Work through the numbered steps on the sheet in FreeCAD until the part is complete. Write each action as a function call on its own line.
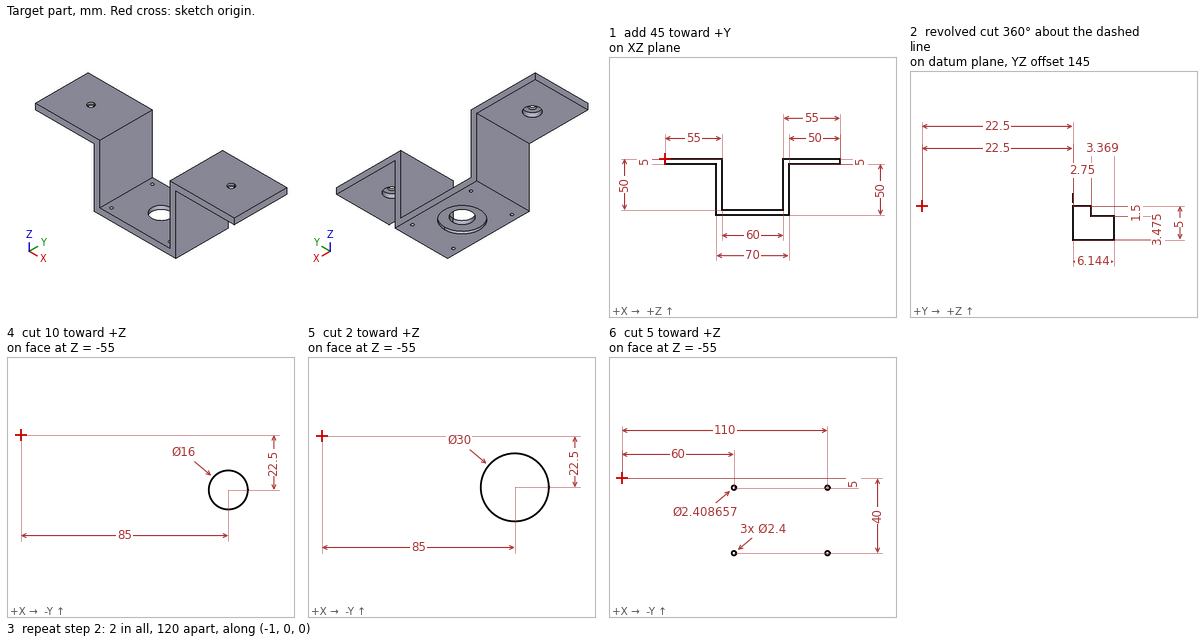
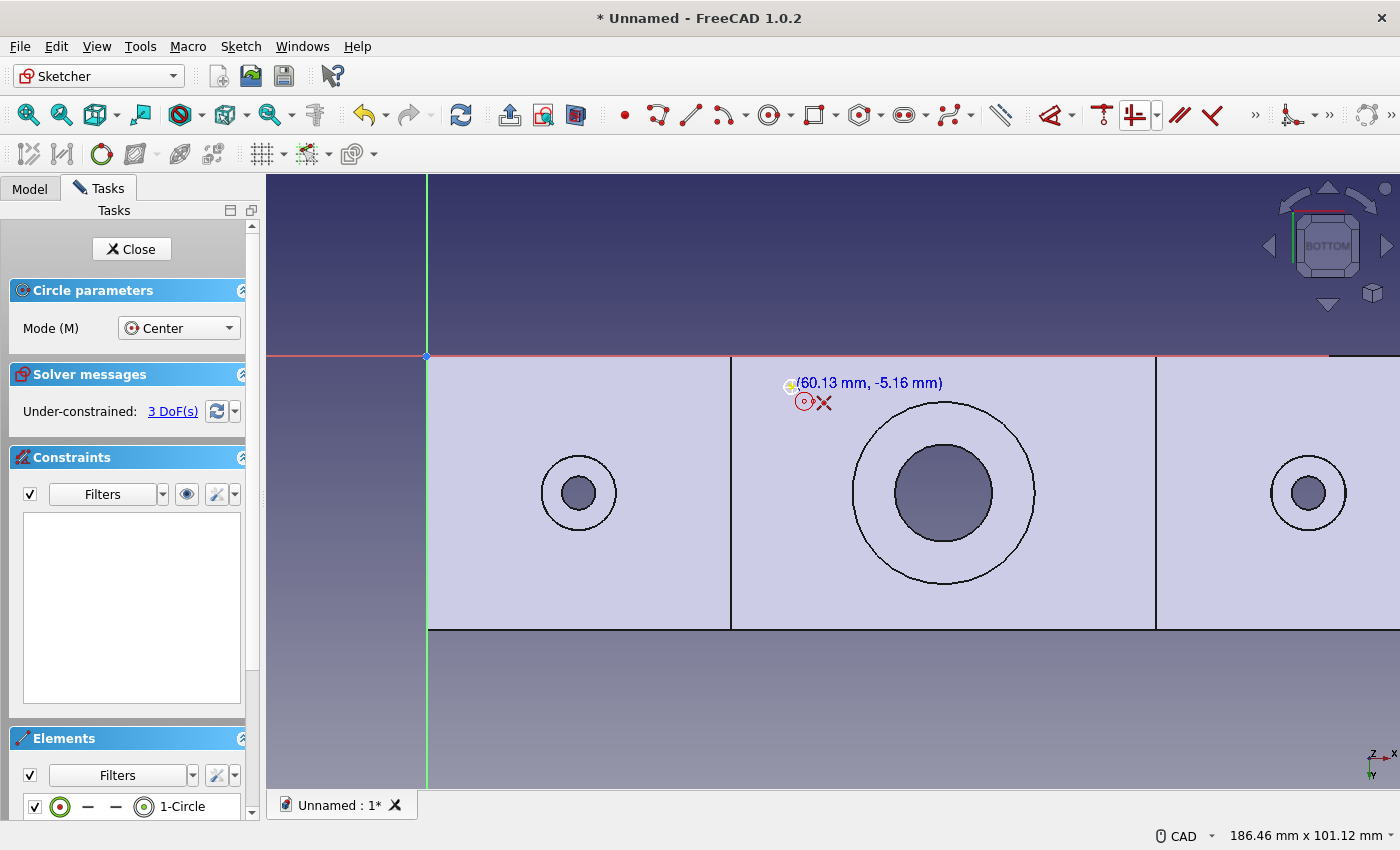
scroll(792, 599, up, 6)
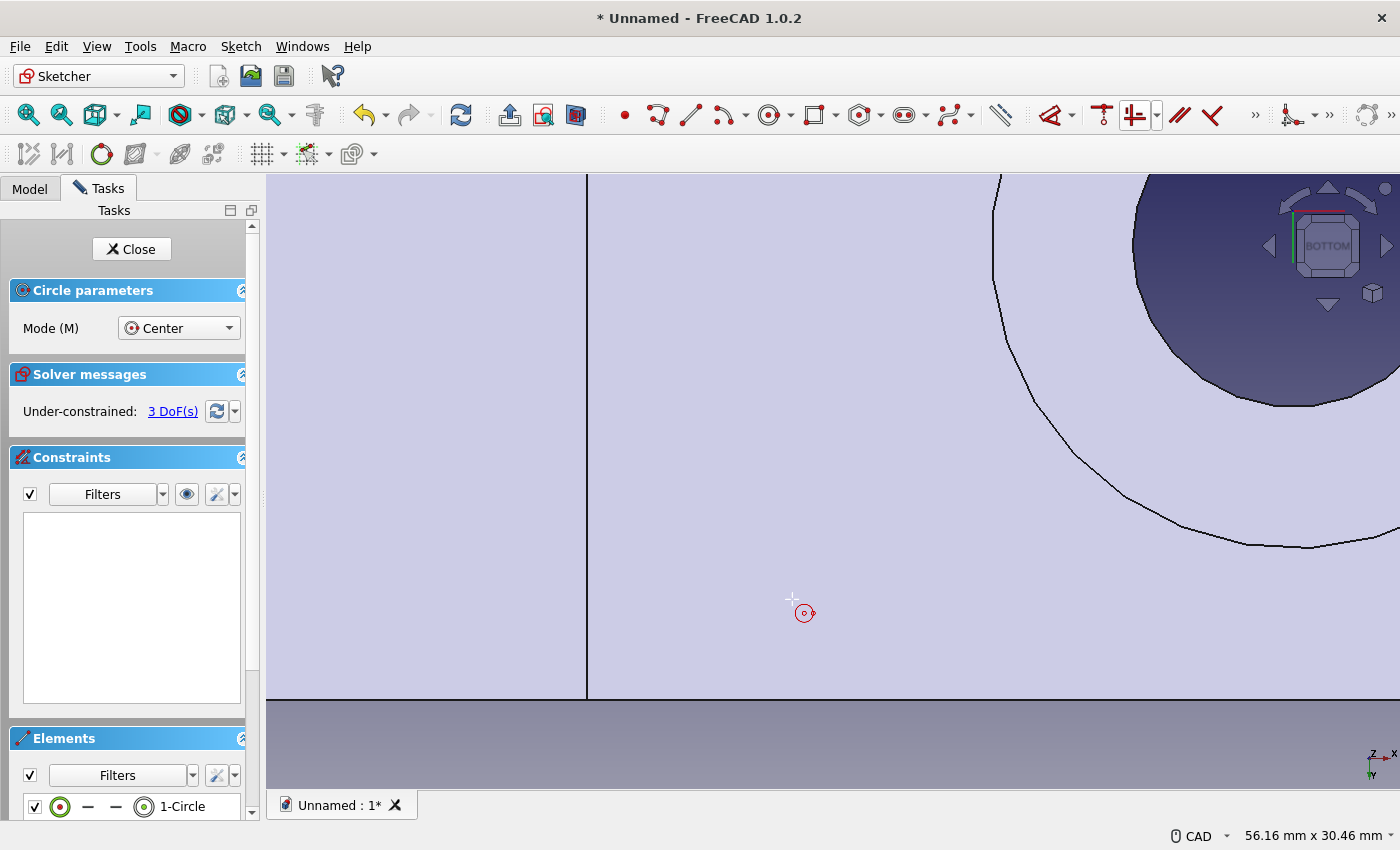
click(789, 599)
click(806, 582)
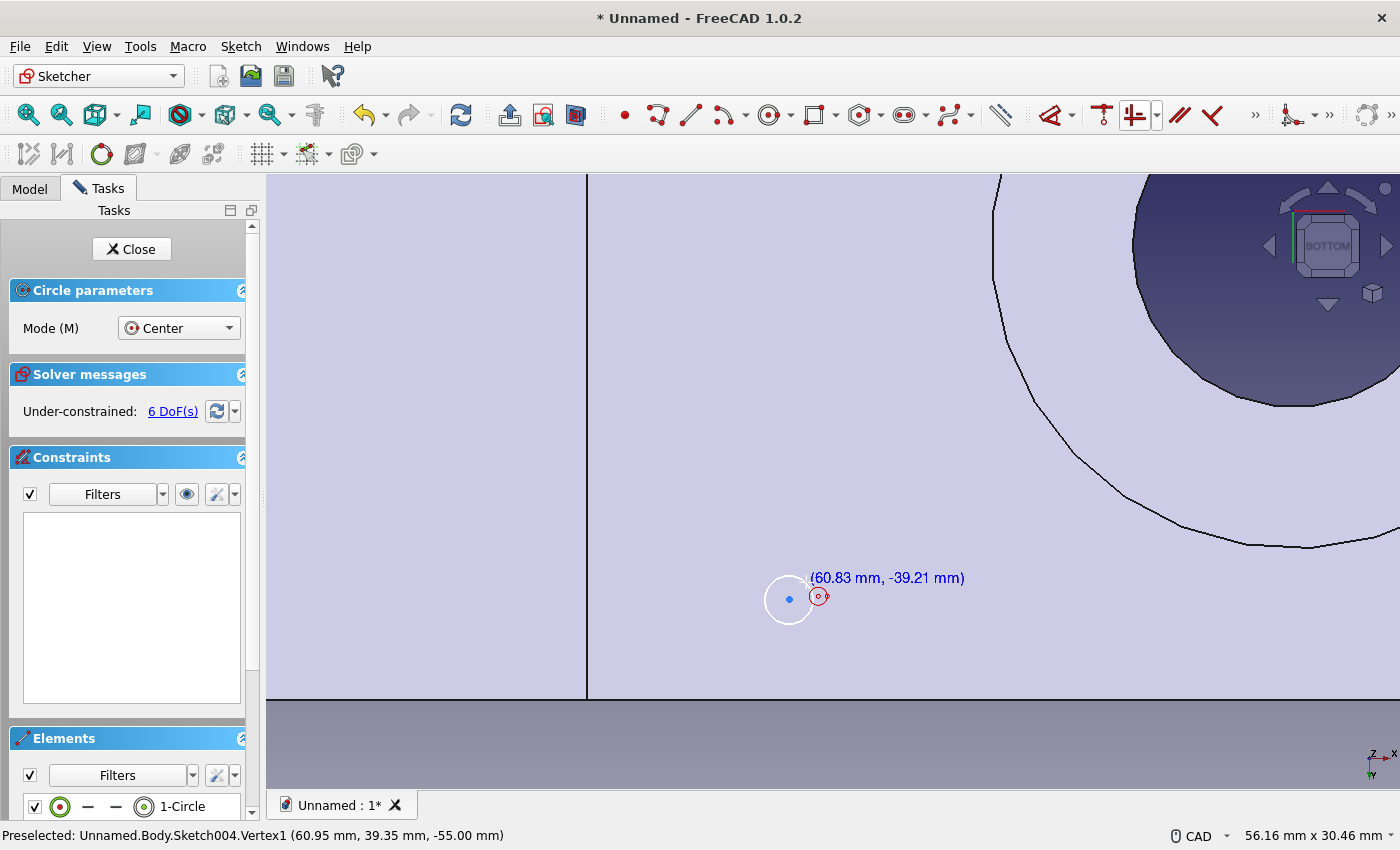
scroll(792, 600, down, 6)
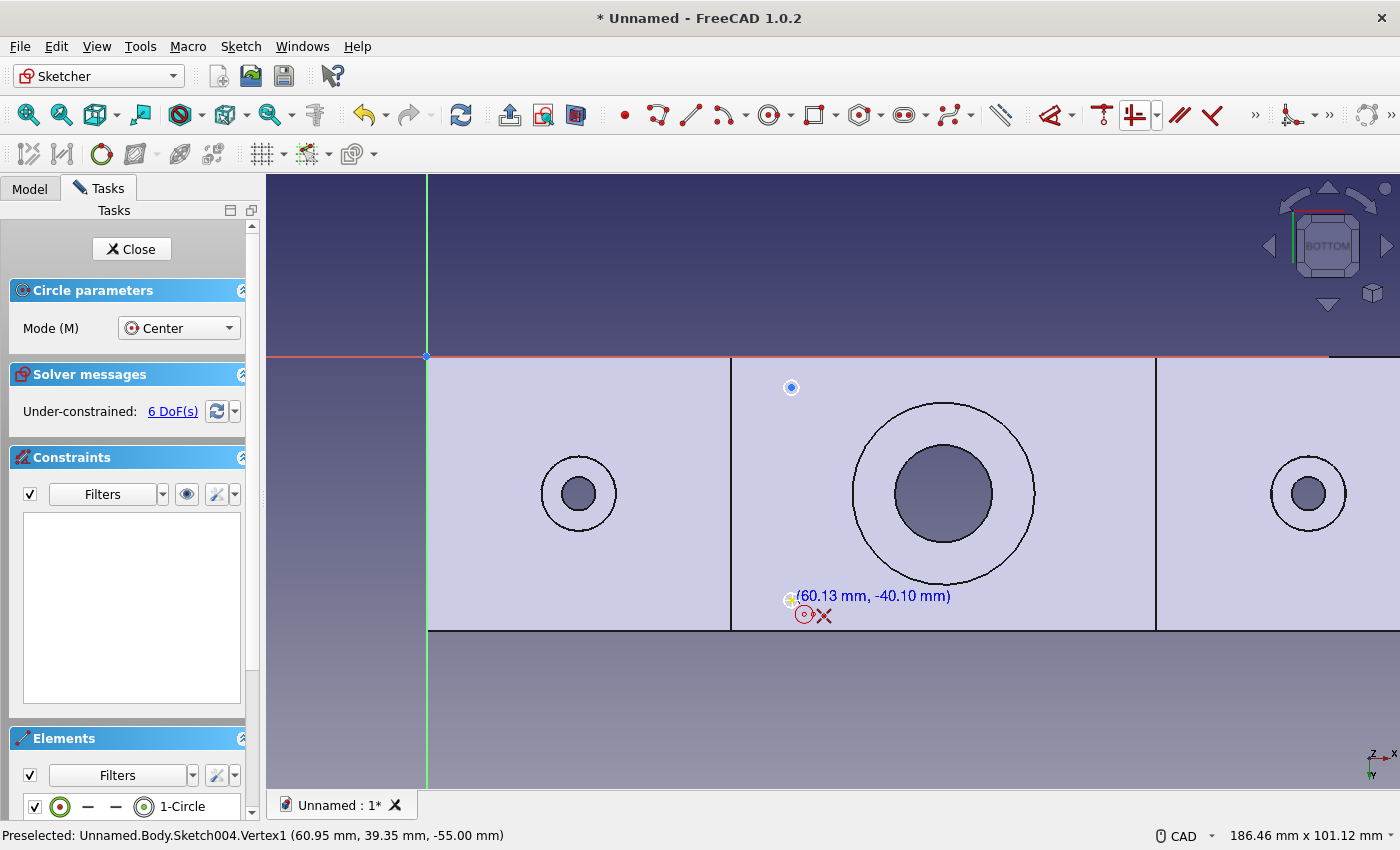
scroll(1096, 387, up, 6)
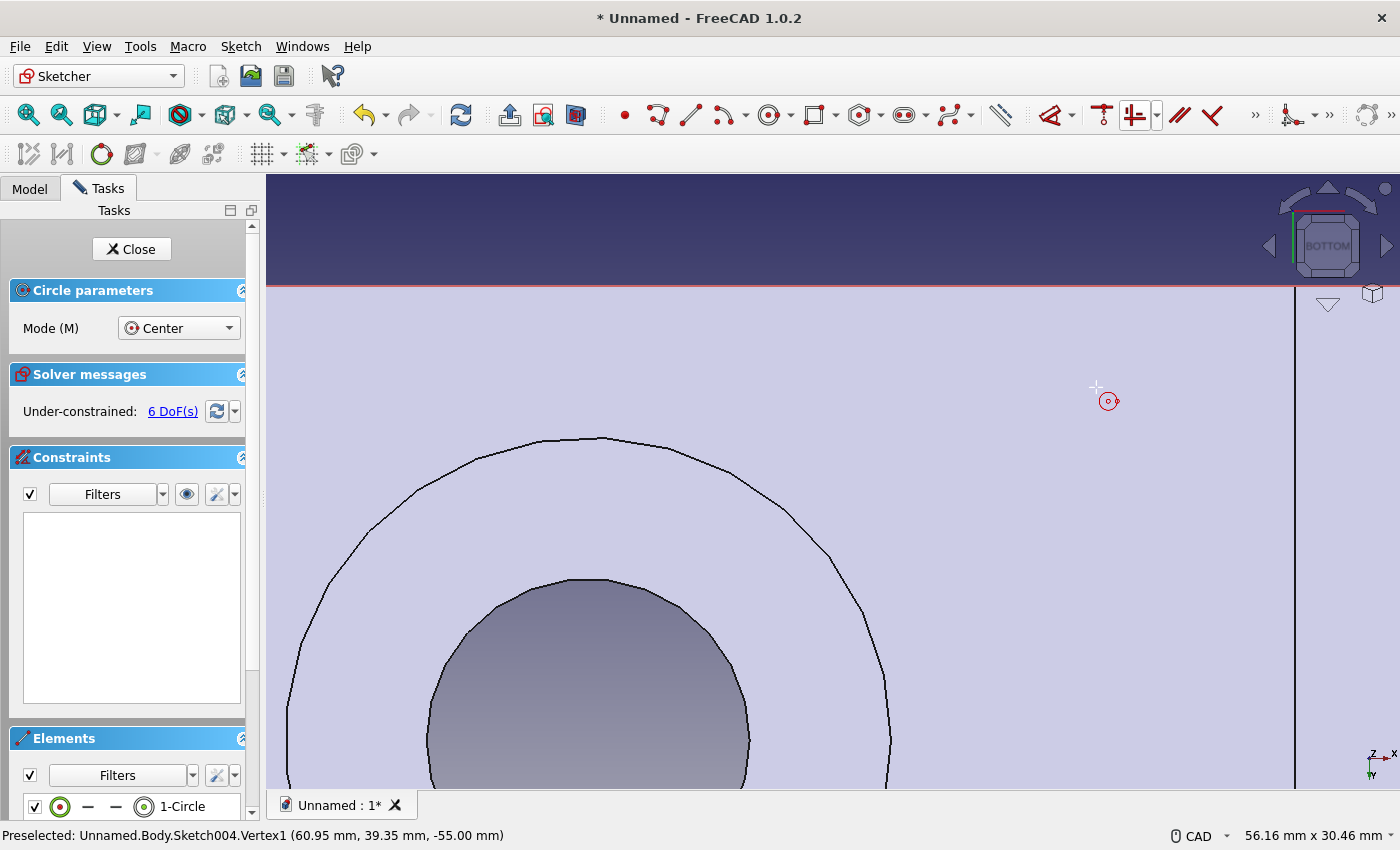
click(1093, 387)
click(1110, 370)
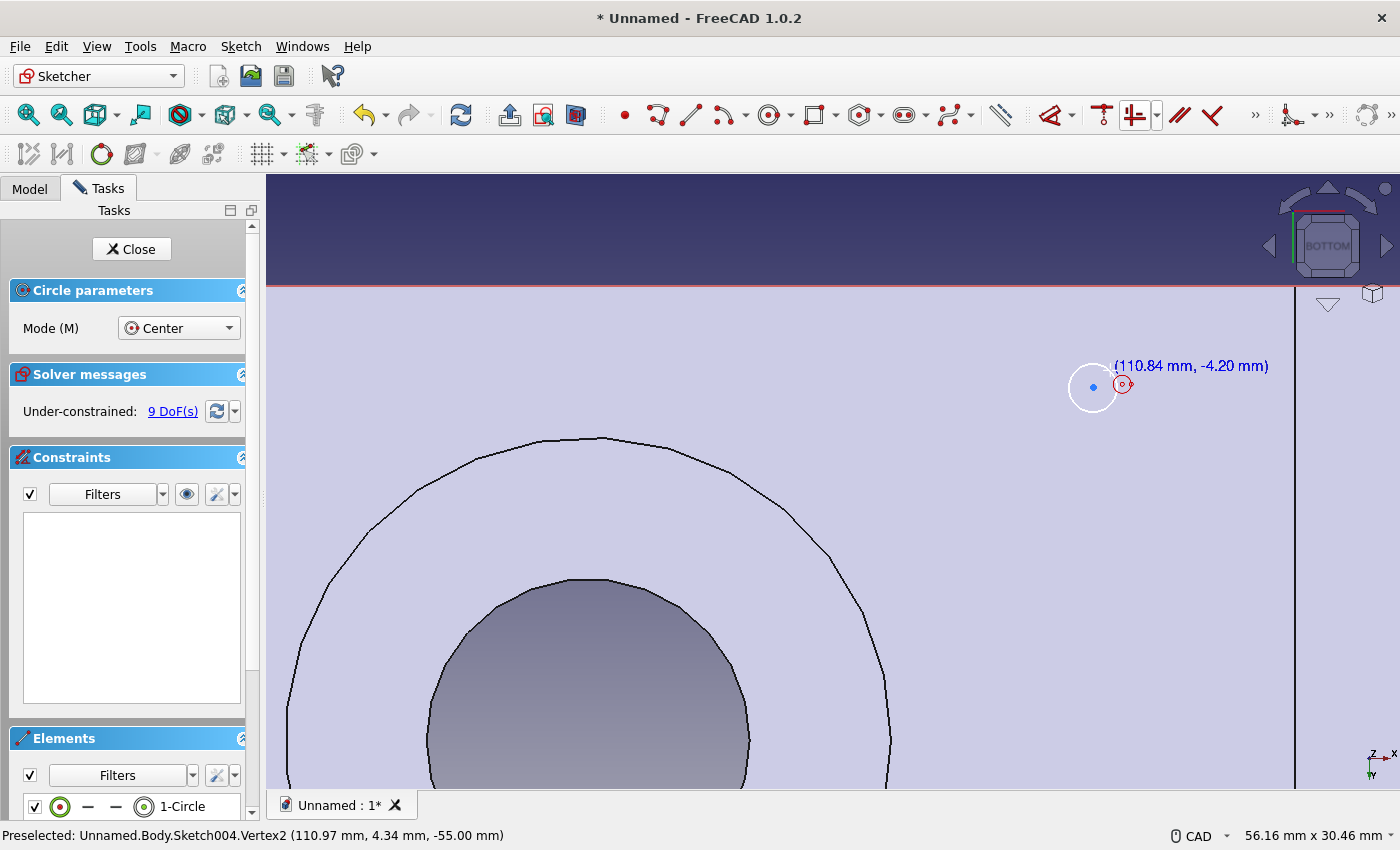
scroll(1096, 386, down, 6)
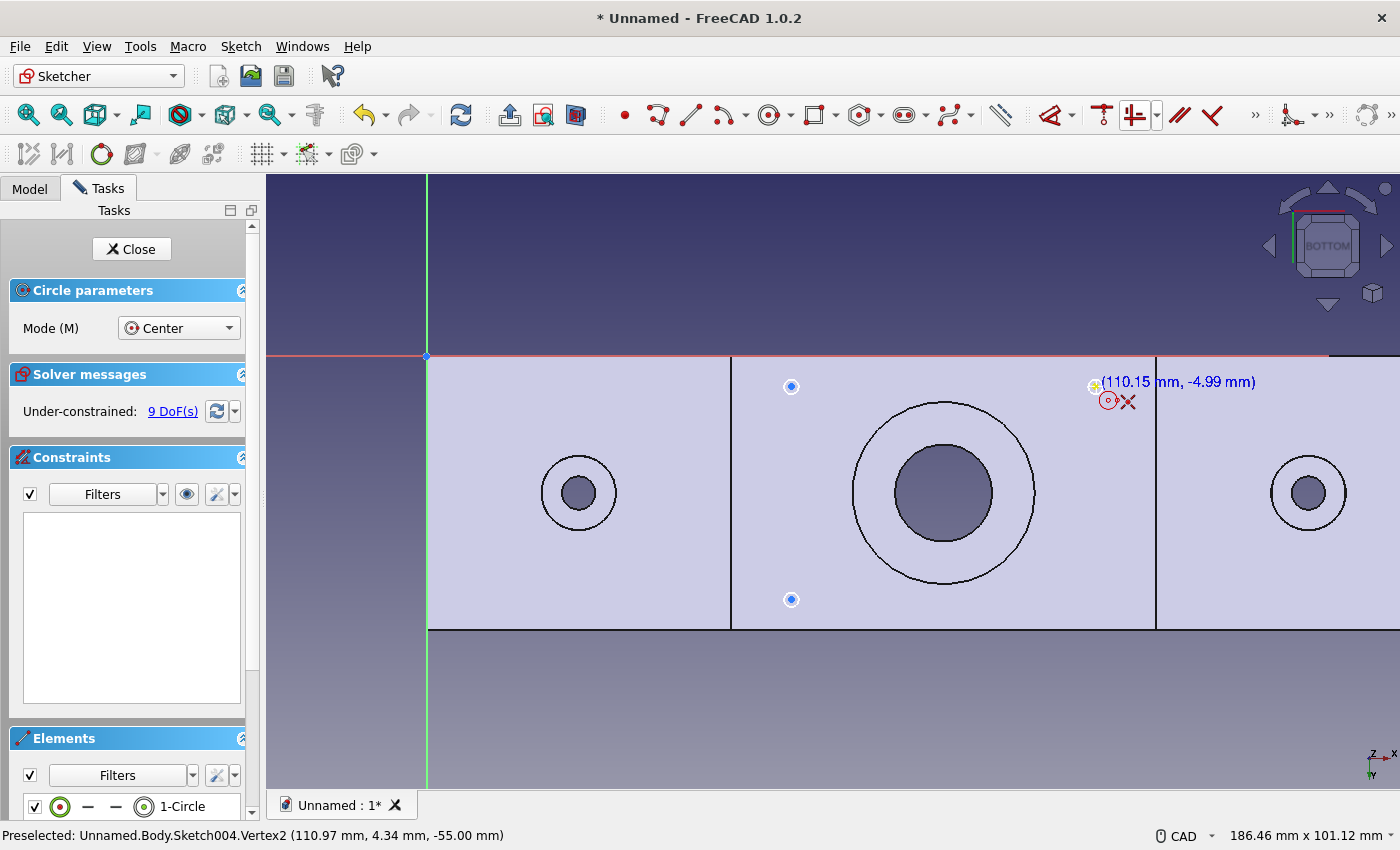
scroll(1096, 599, up, 6)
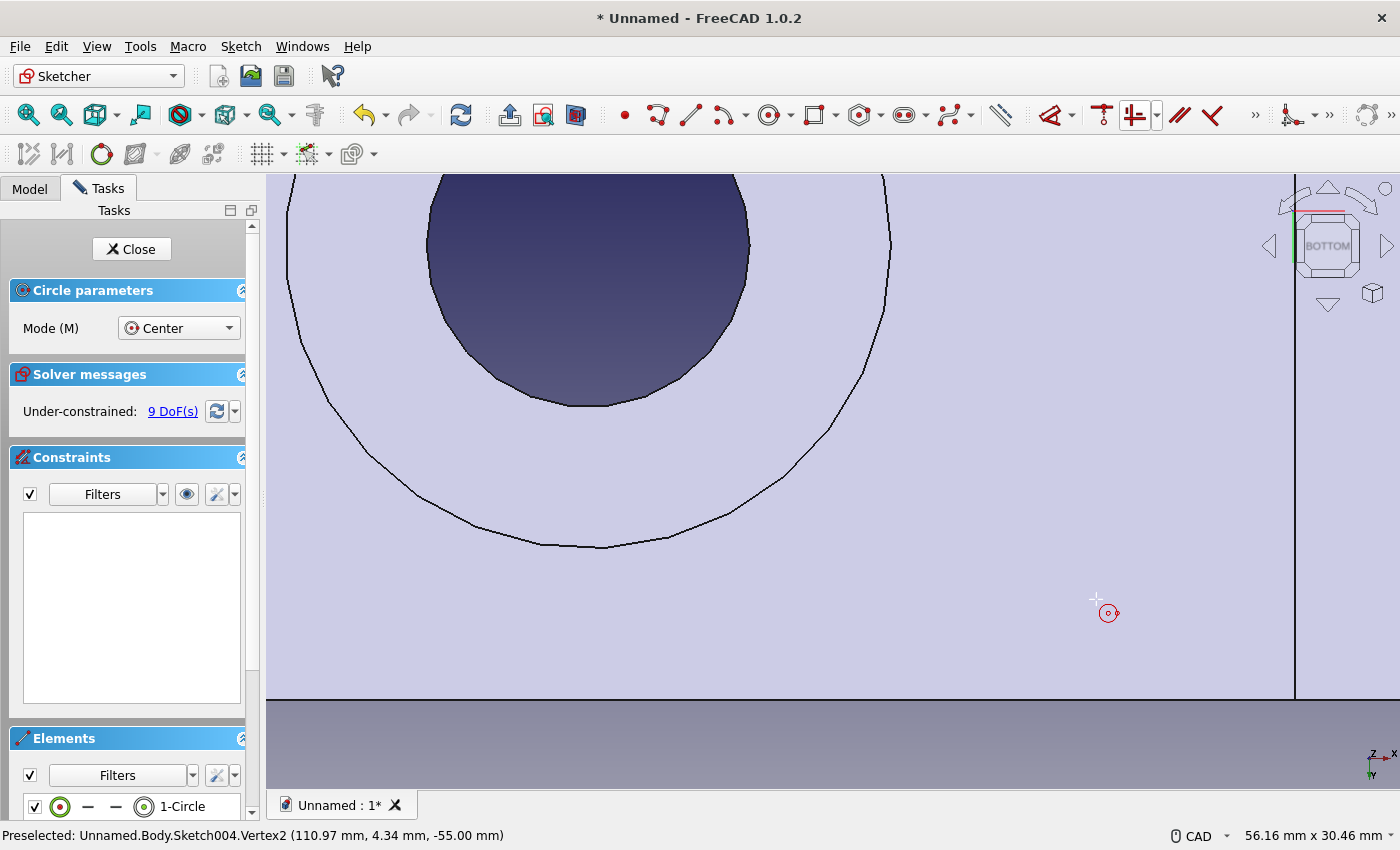
click(1093, 599)
click(1110, 582)
key(Escape)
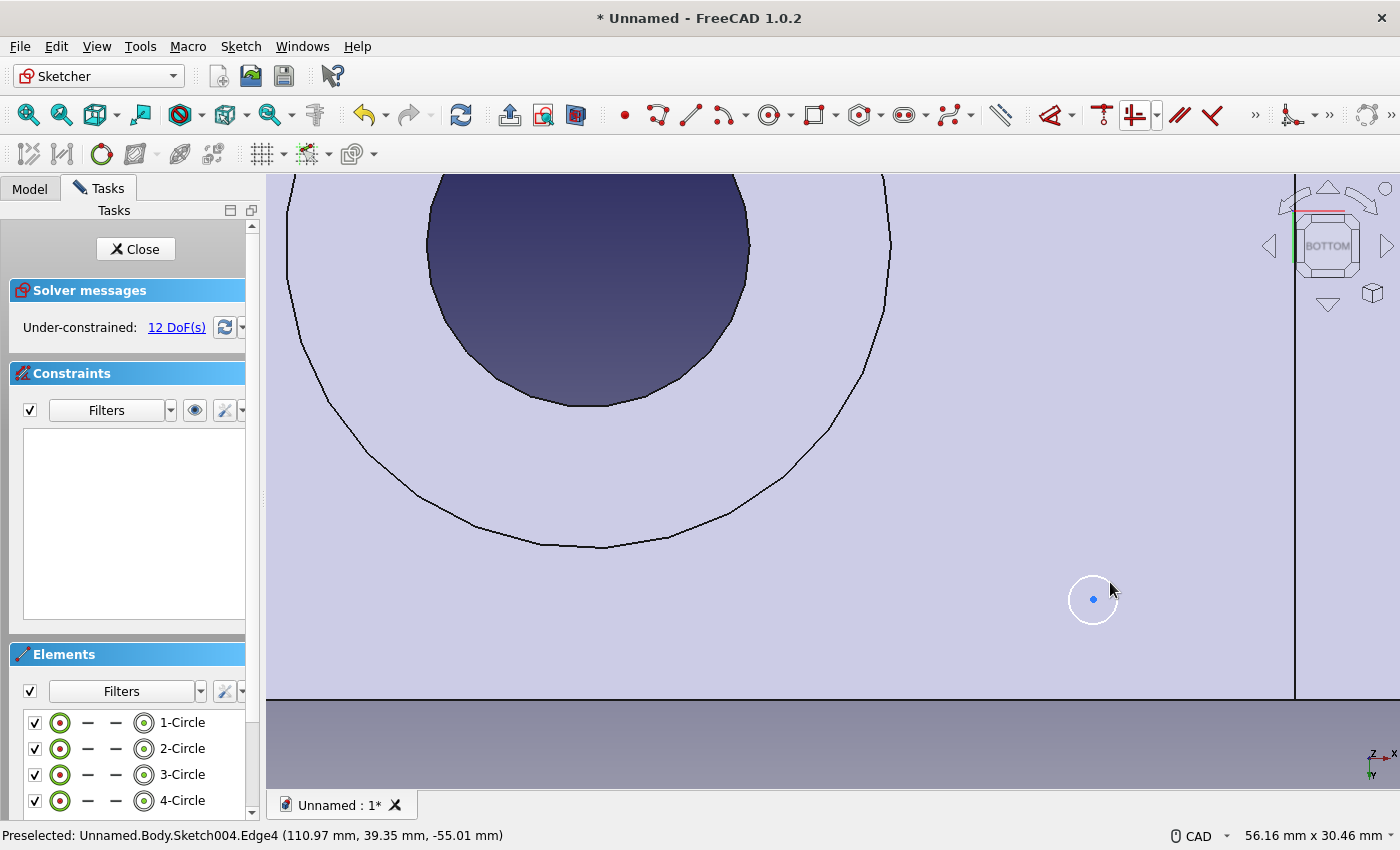
scroll(1096, 600, down, 6)